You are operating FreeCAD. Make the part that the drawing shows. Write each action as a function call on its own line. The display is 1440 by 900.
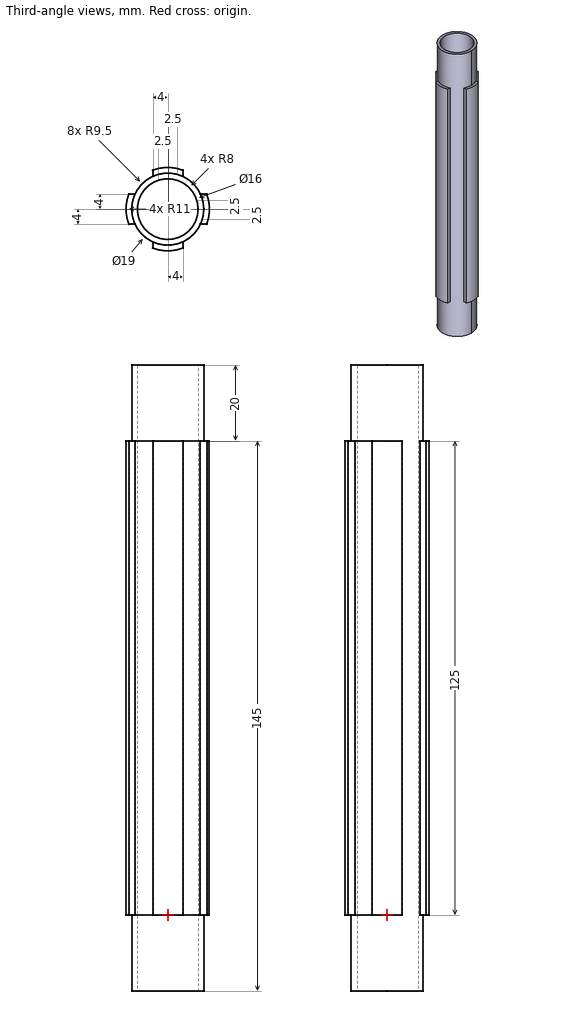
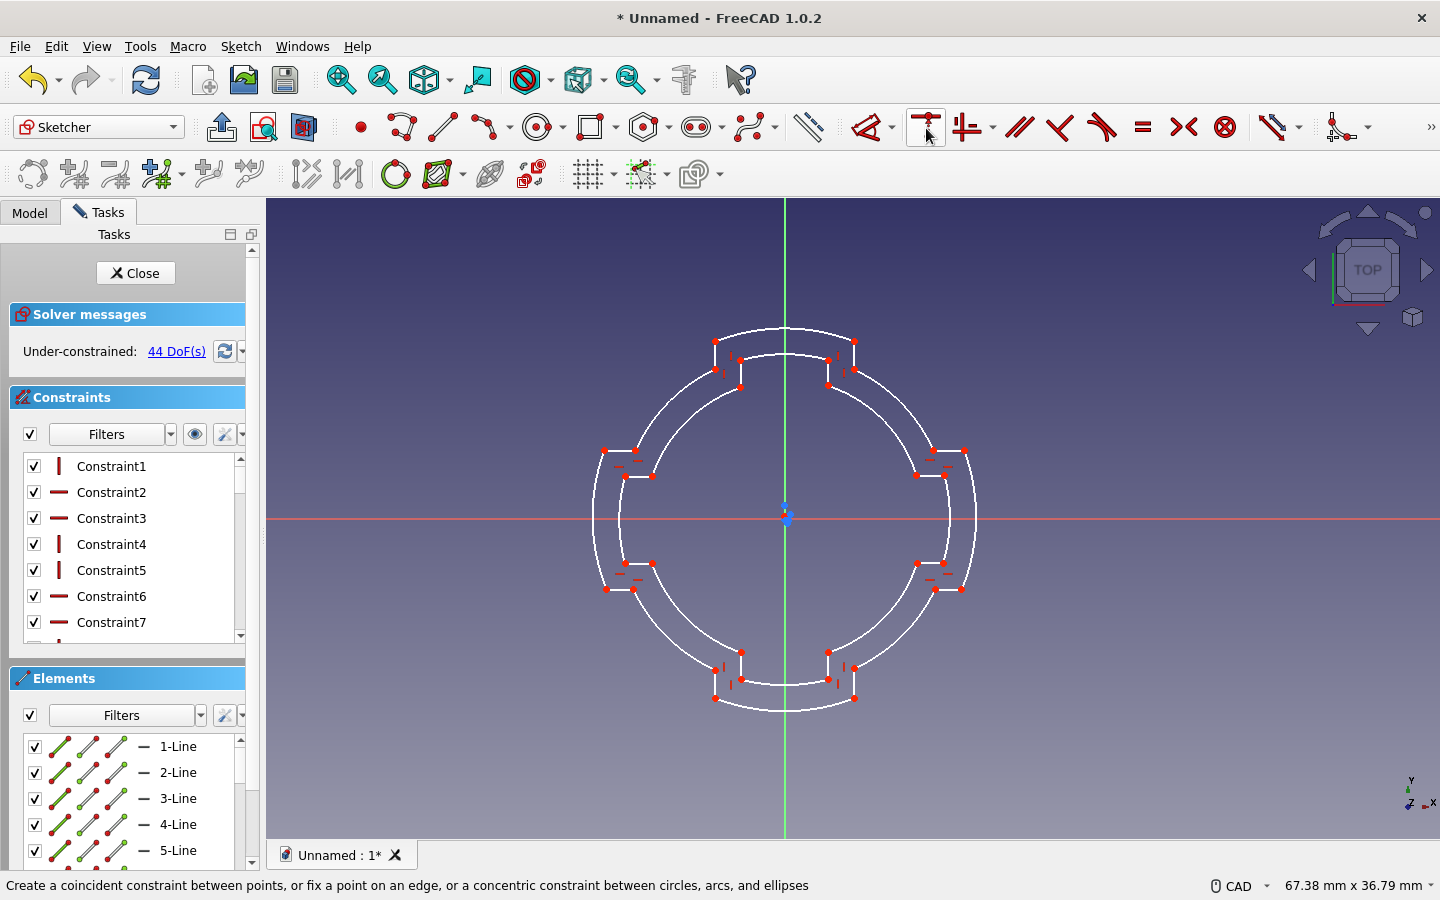
click(686, 387)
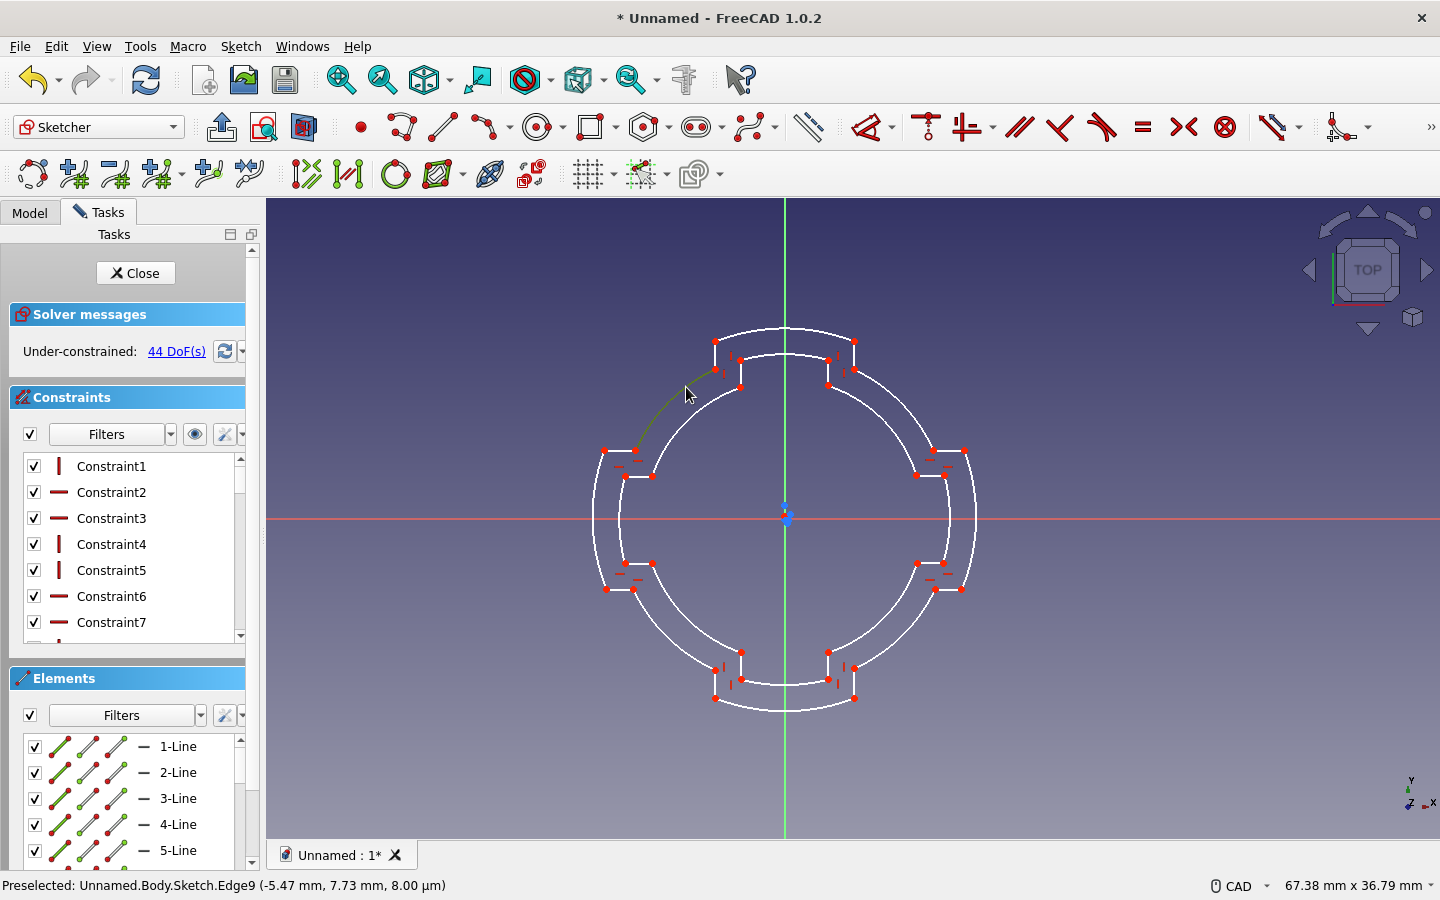
click(863, 635)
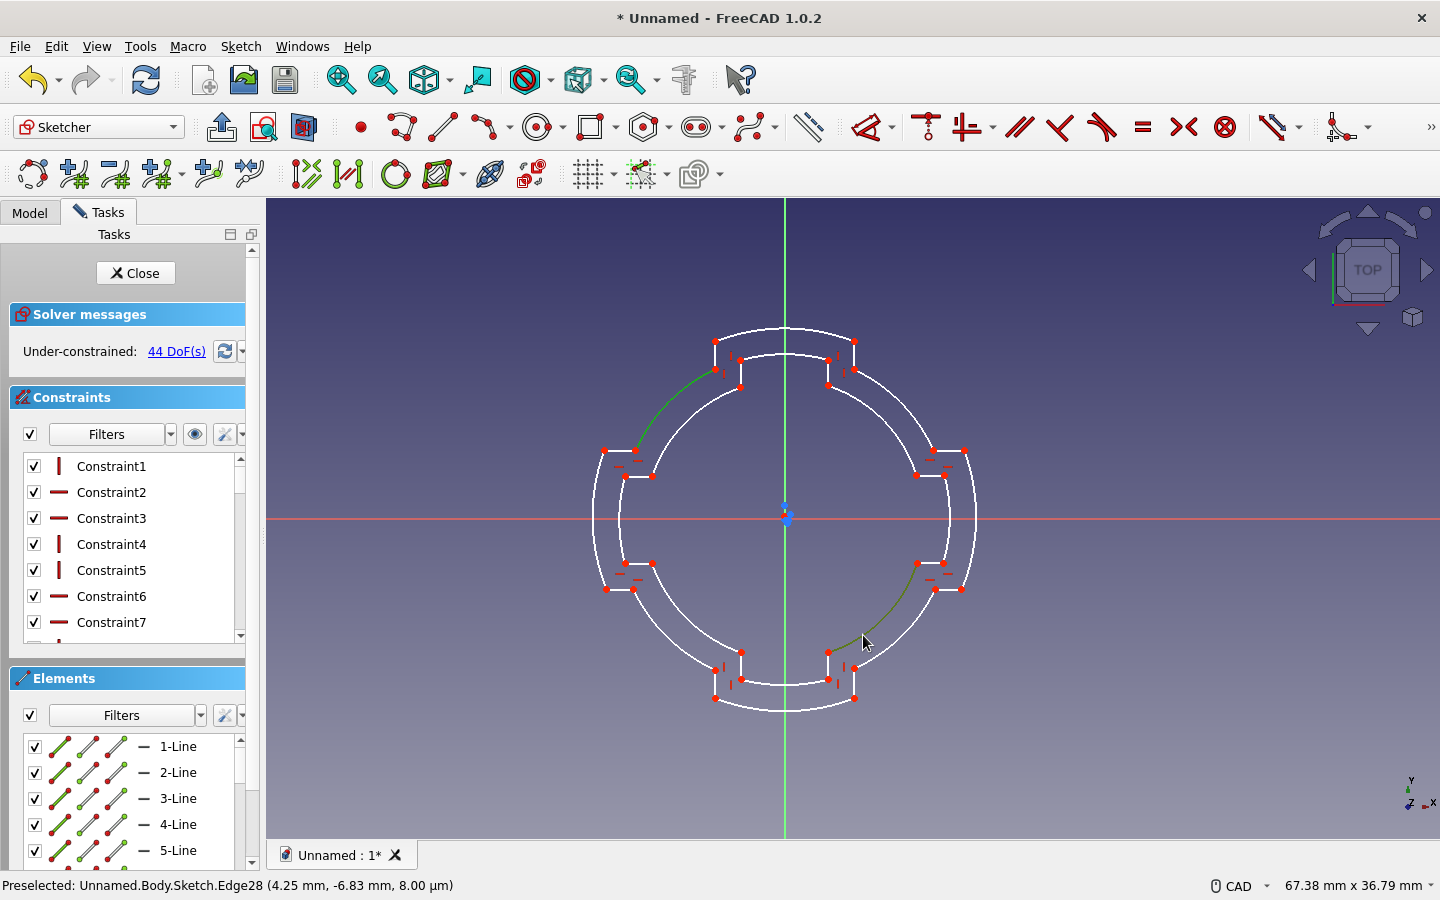
click(926, 128)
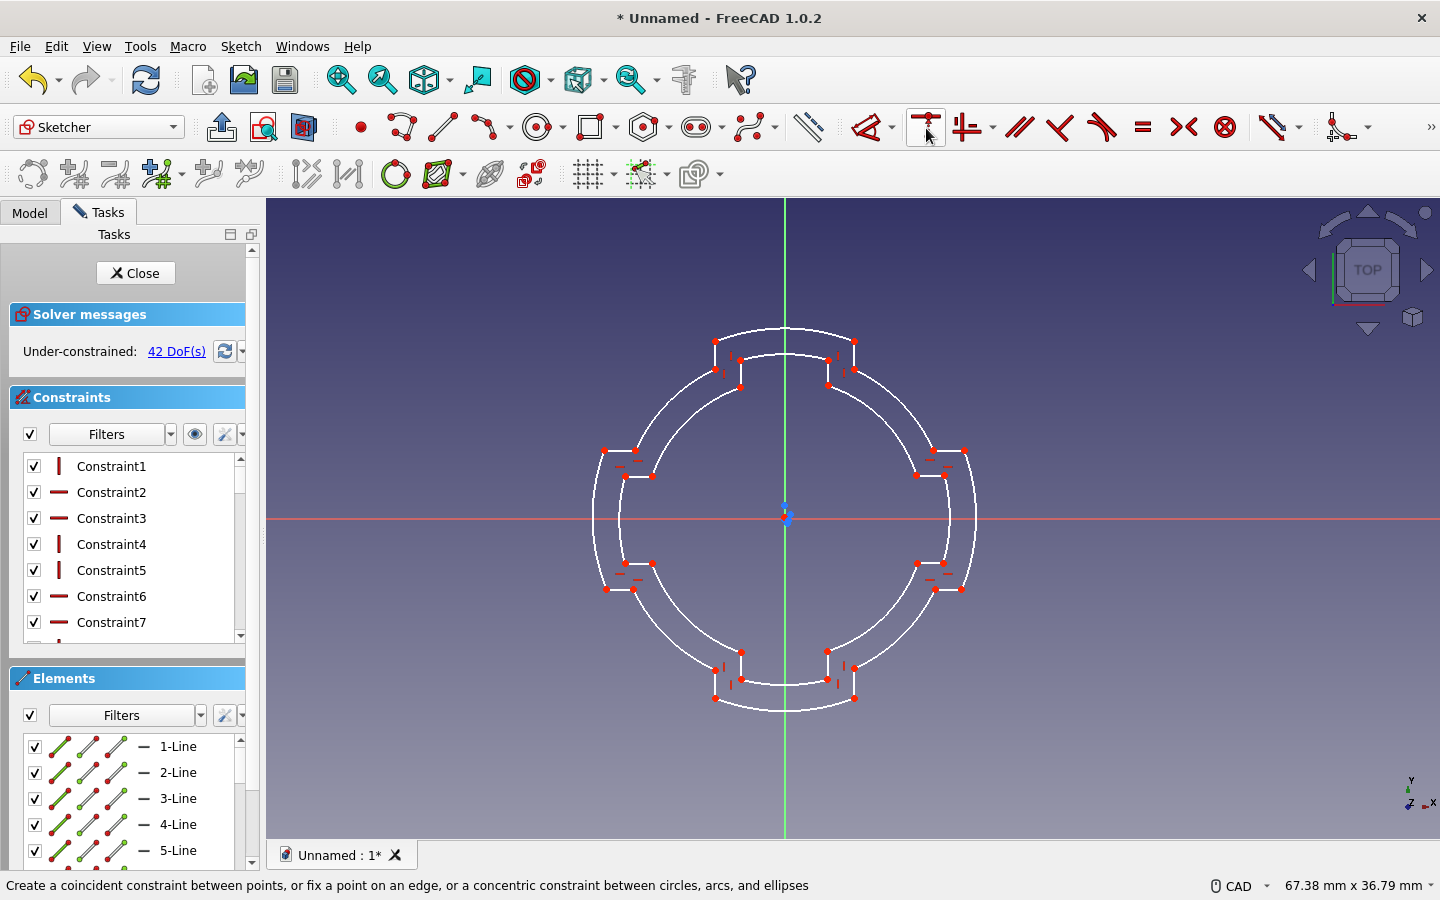
click(686, 387)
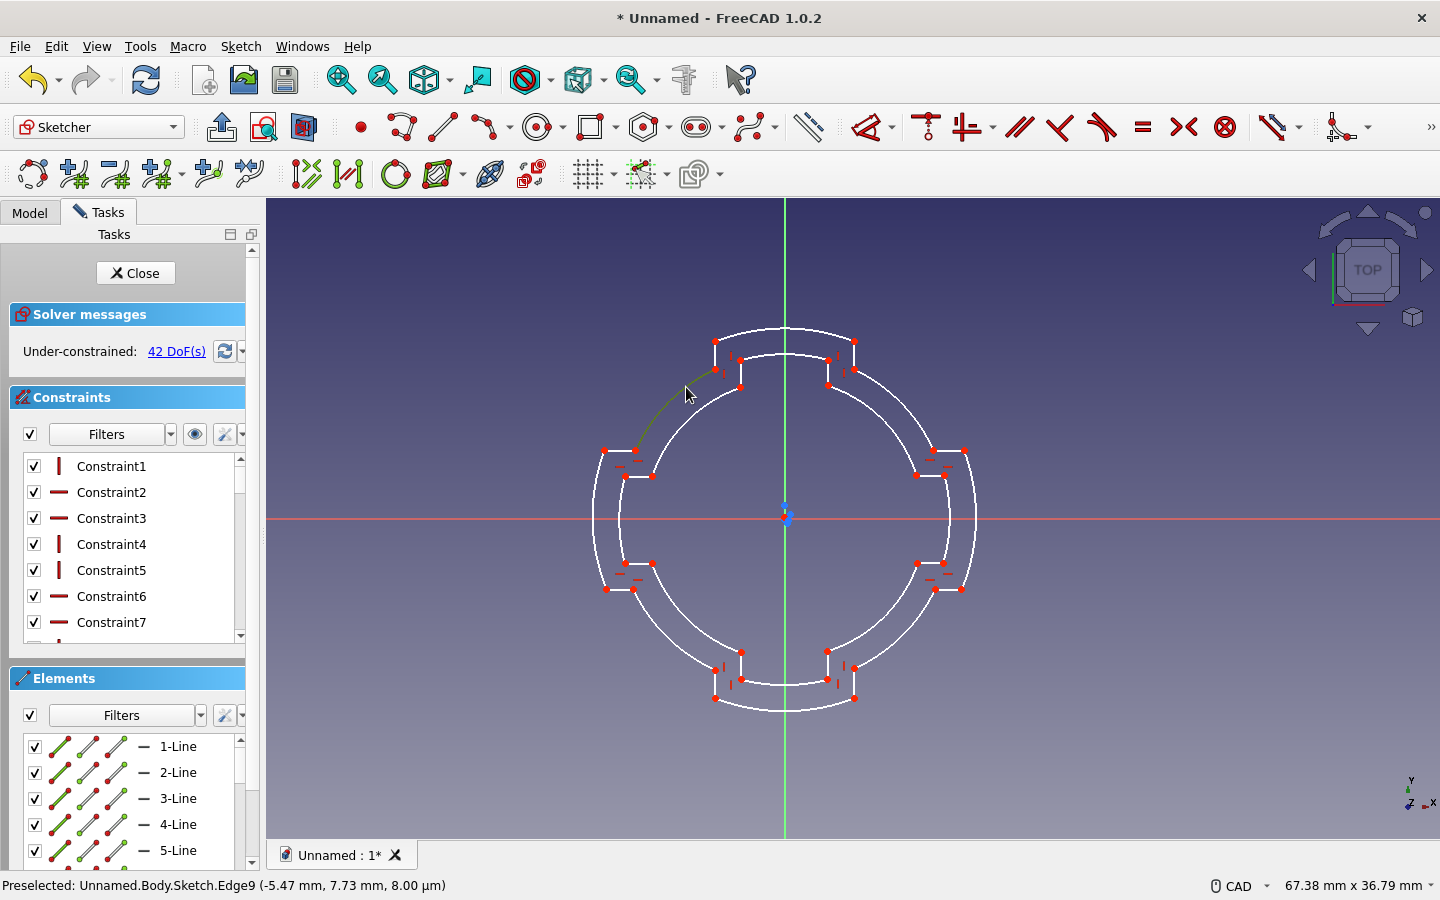
click(767, 684)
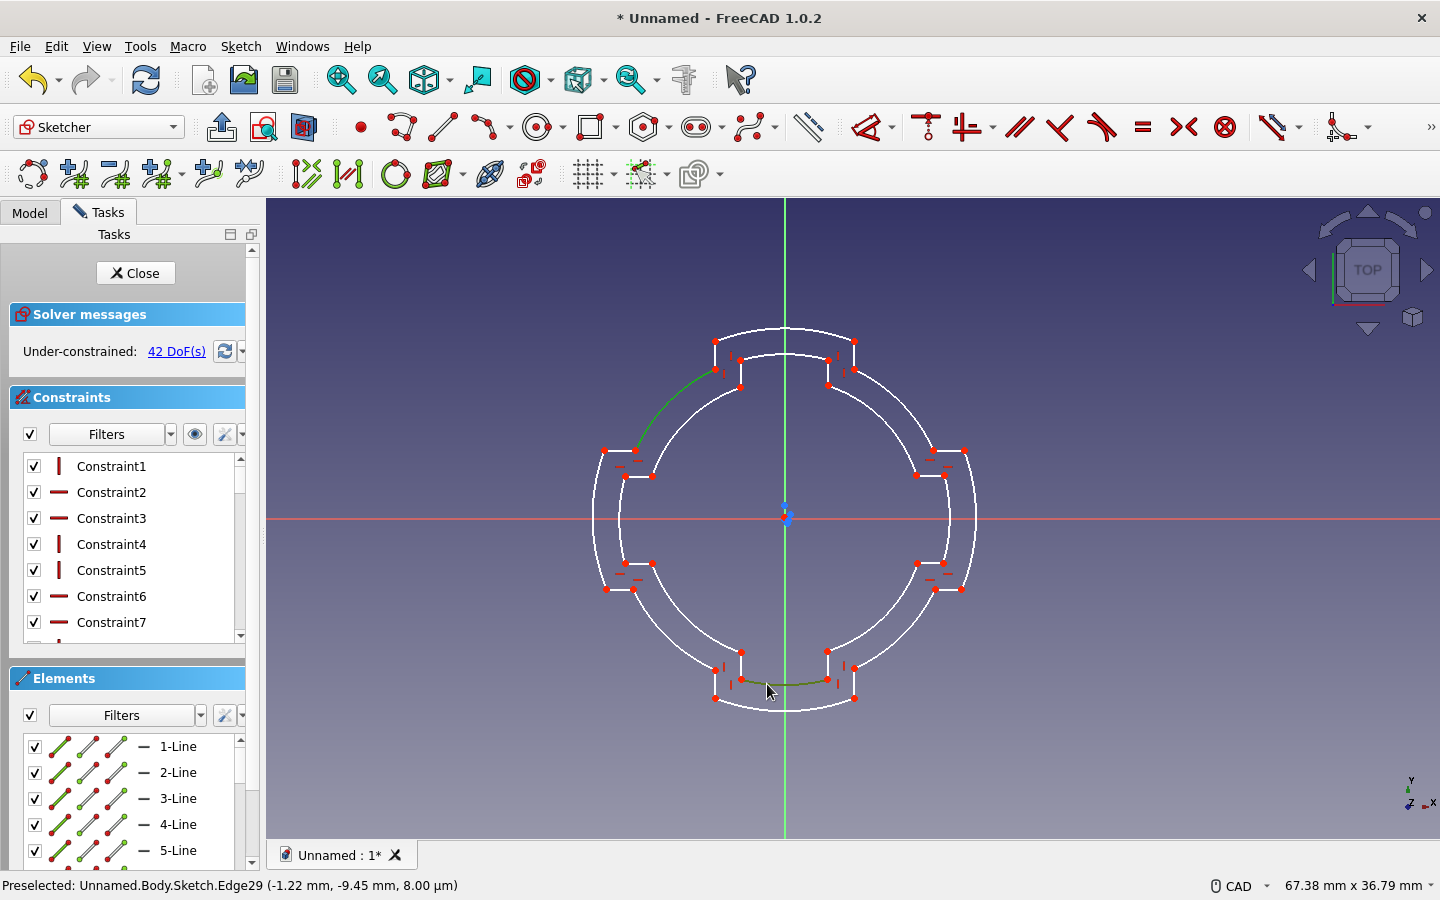
click(926, 128)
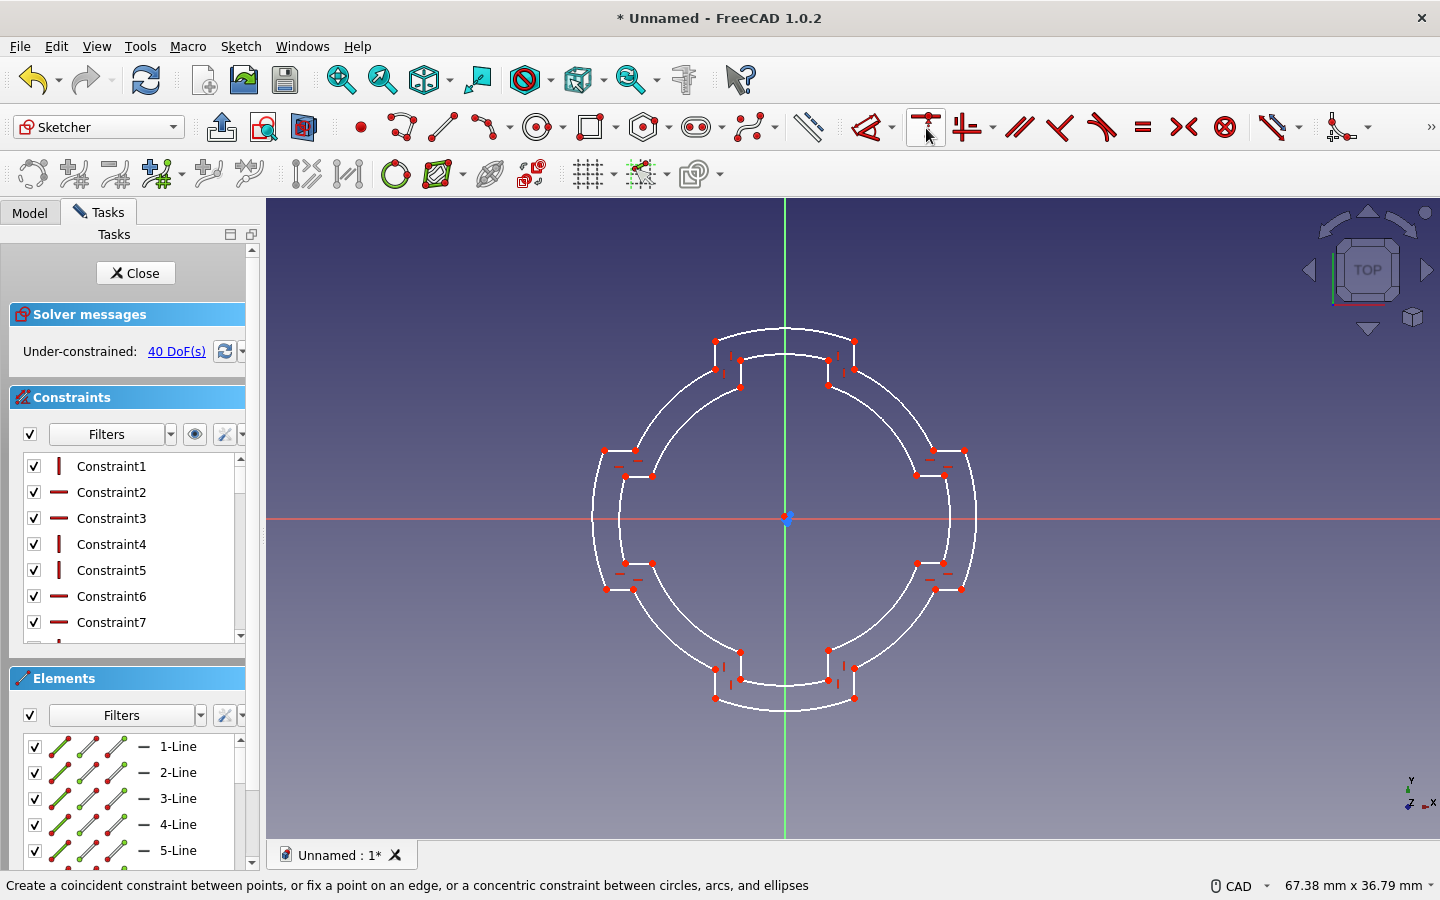
click(686, 387)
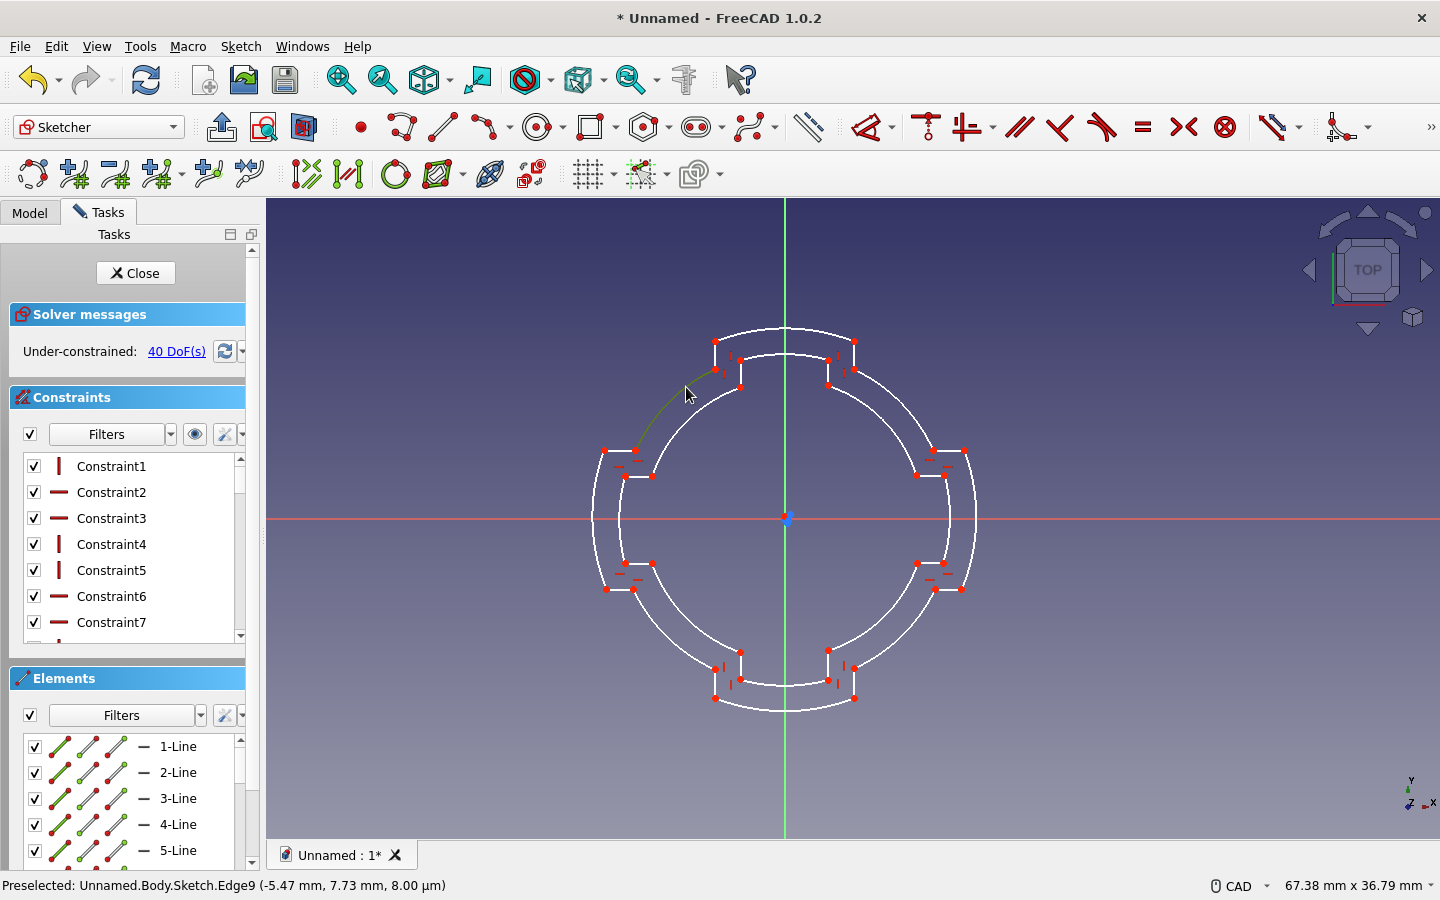
click(670, 598)